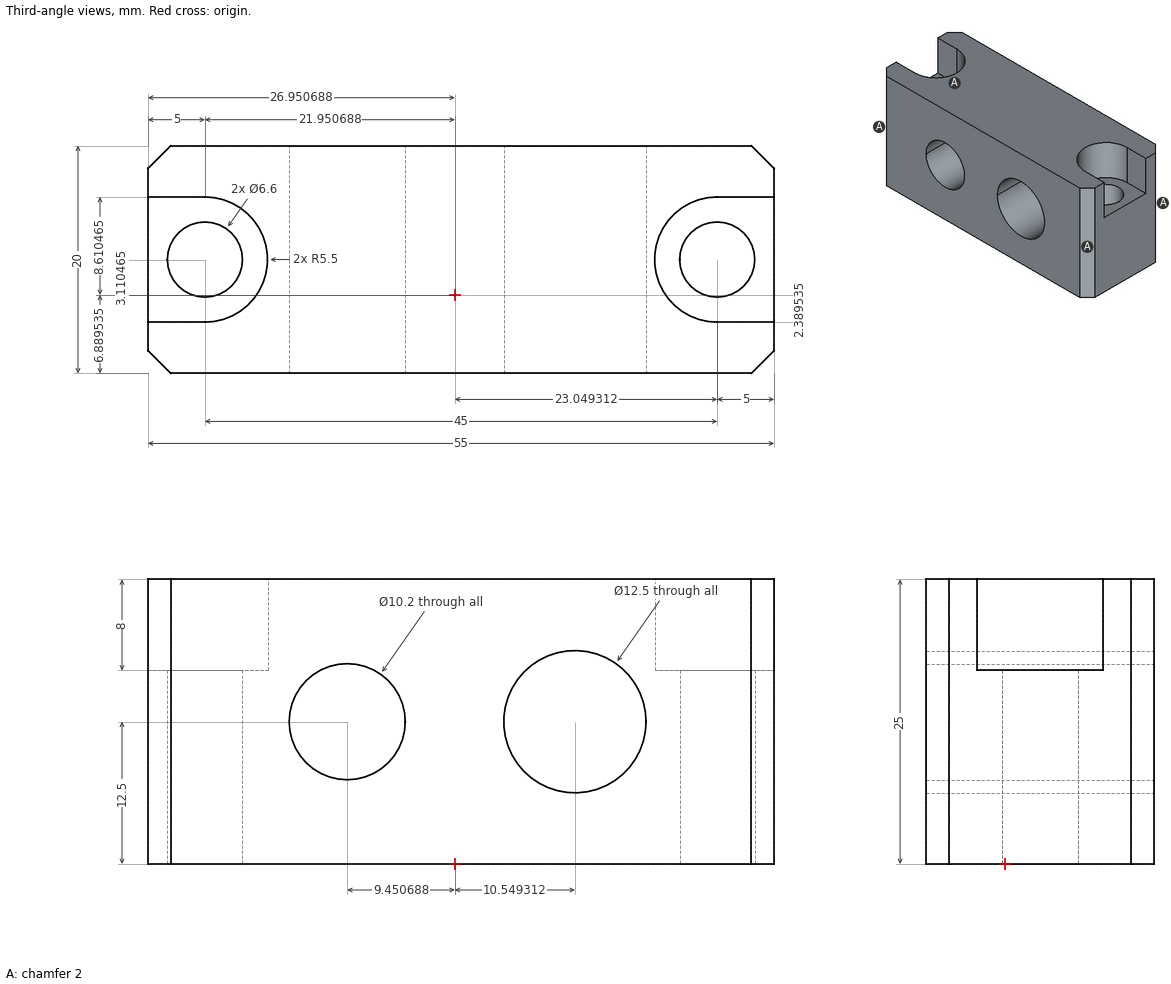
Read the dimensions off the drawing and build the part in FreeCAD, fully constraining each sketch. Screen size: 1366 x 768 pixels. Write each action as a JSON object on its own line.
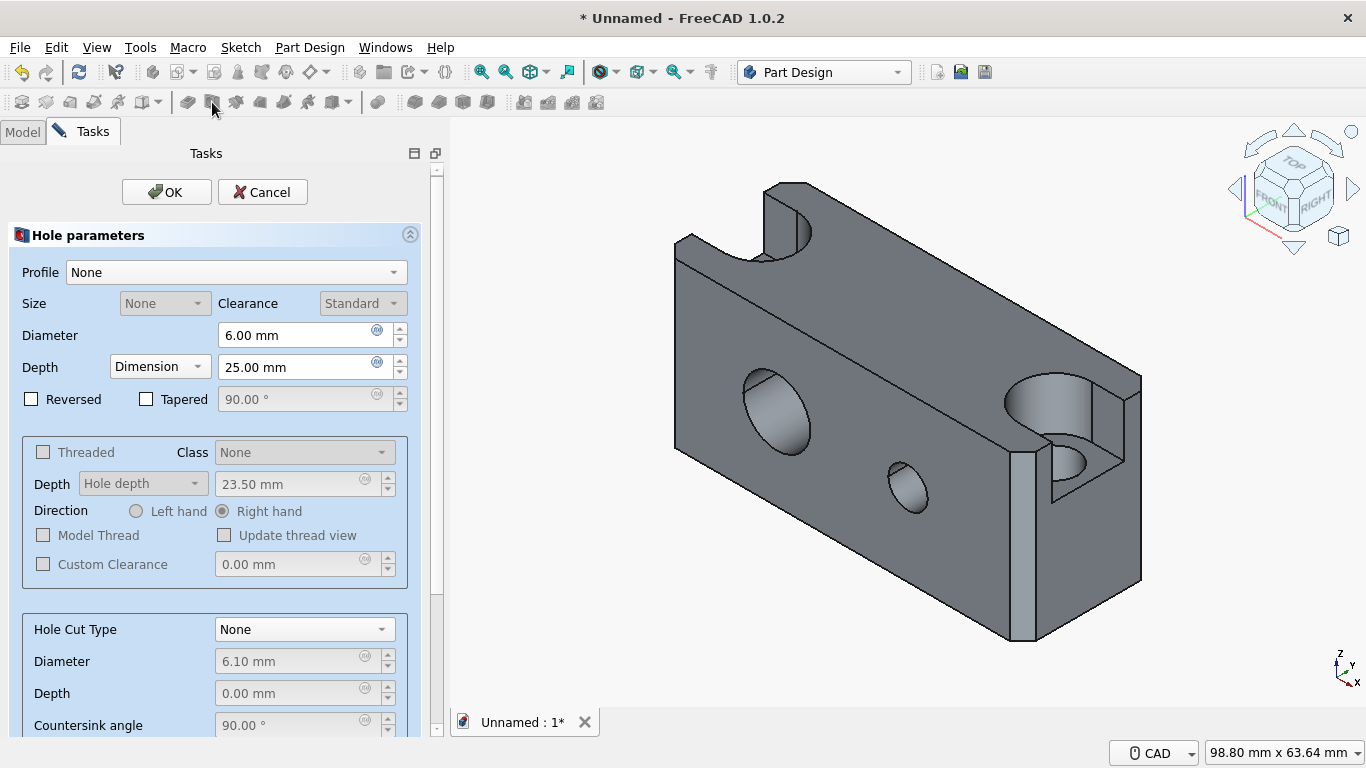
{"action": "triple_click", "coordinate": [305, 335]}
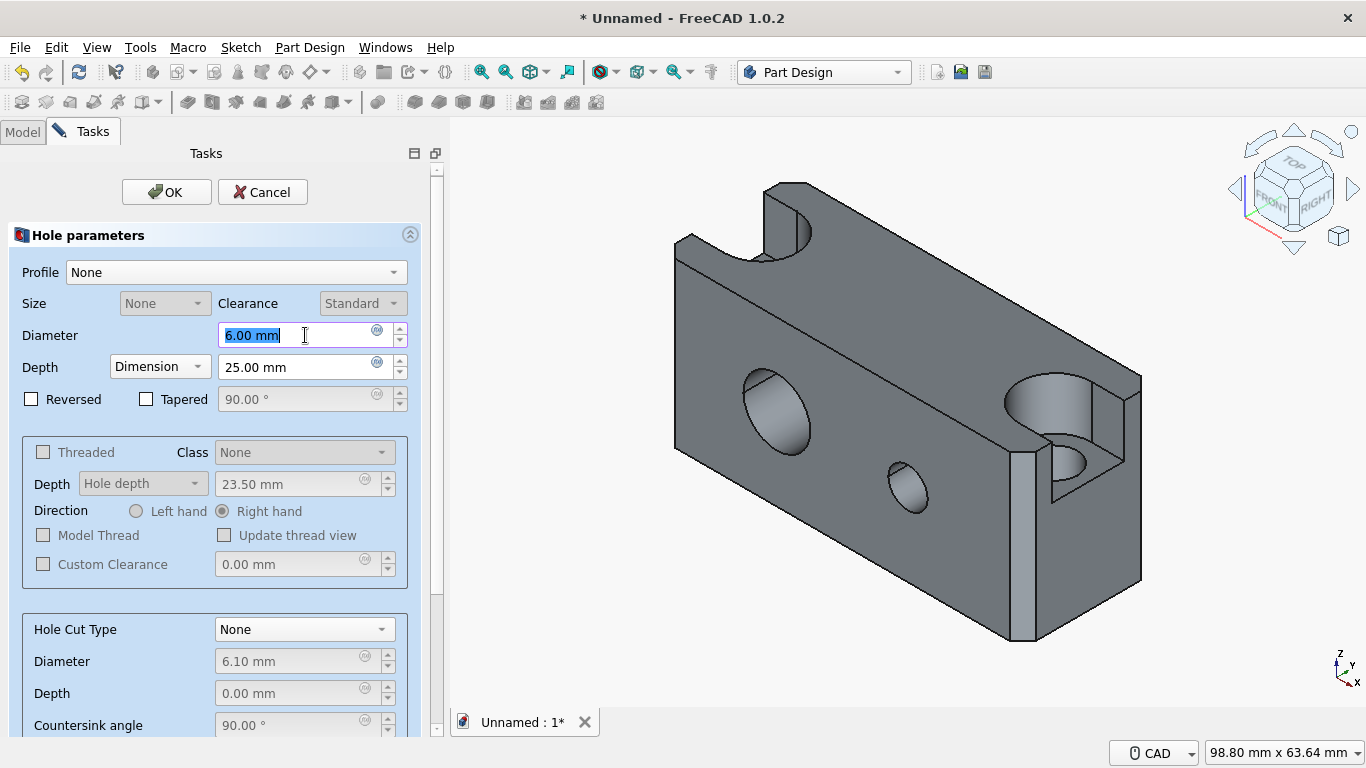
{"action": "type", "text": "12.5"}
{"action": "key", "text": "Tab"}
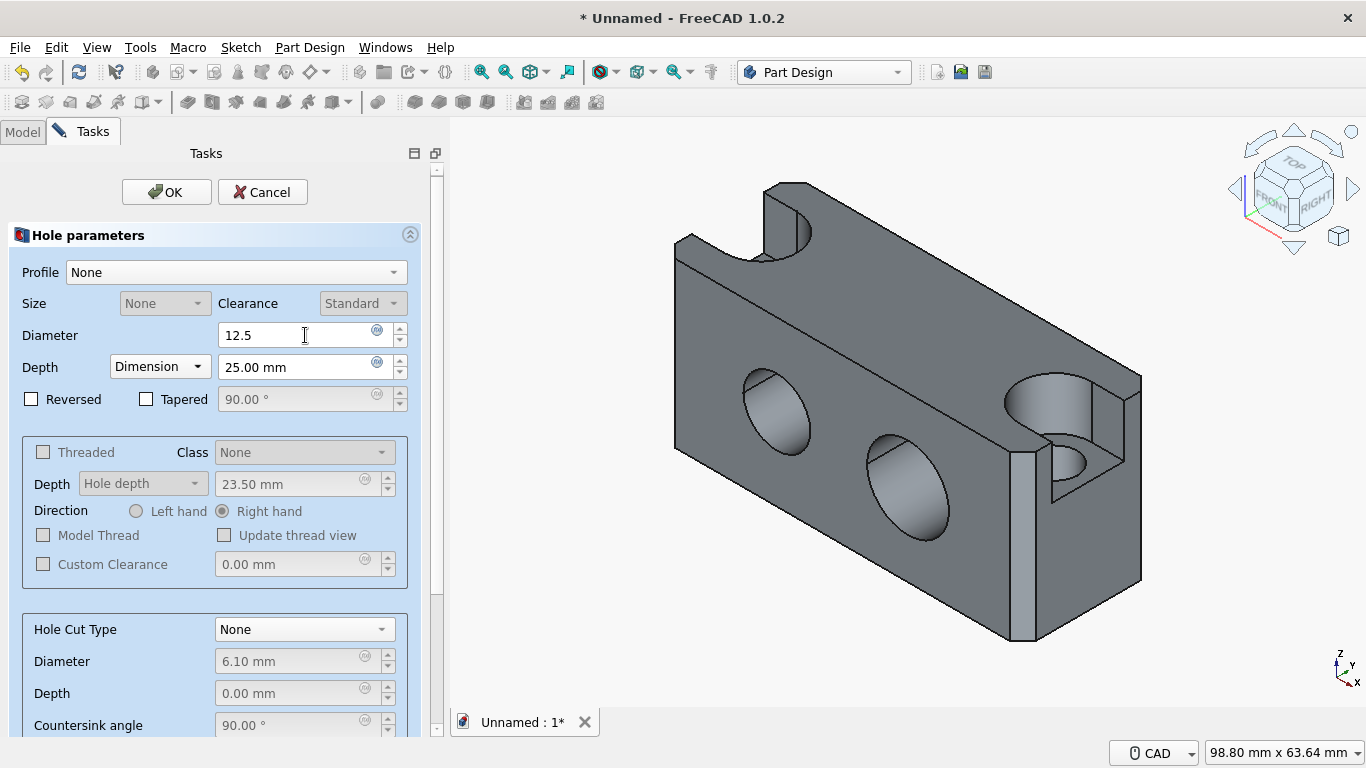
{"action": "left_click", "coordinate": [161, 366]}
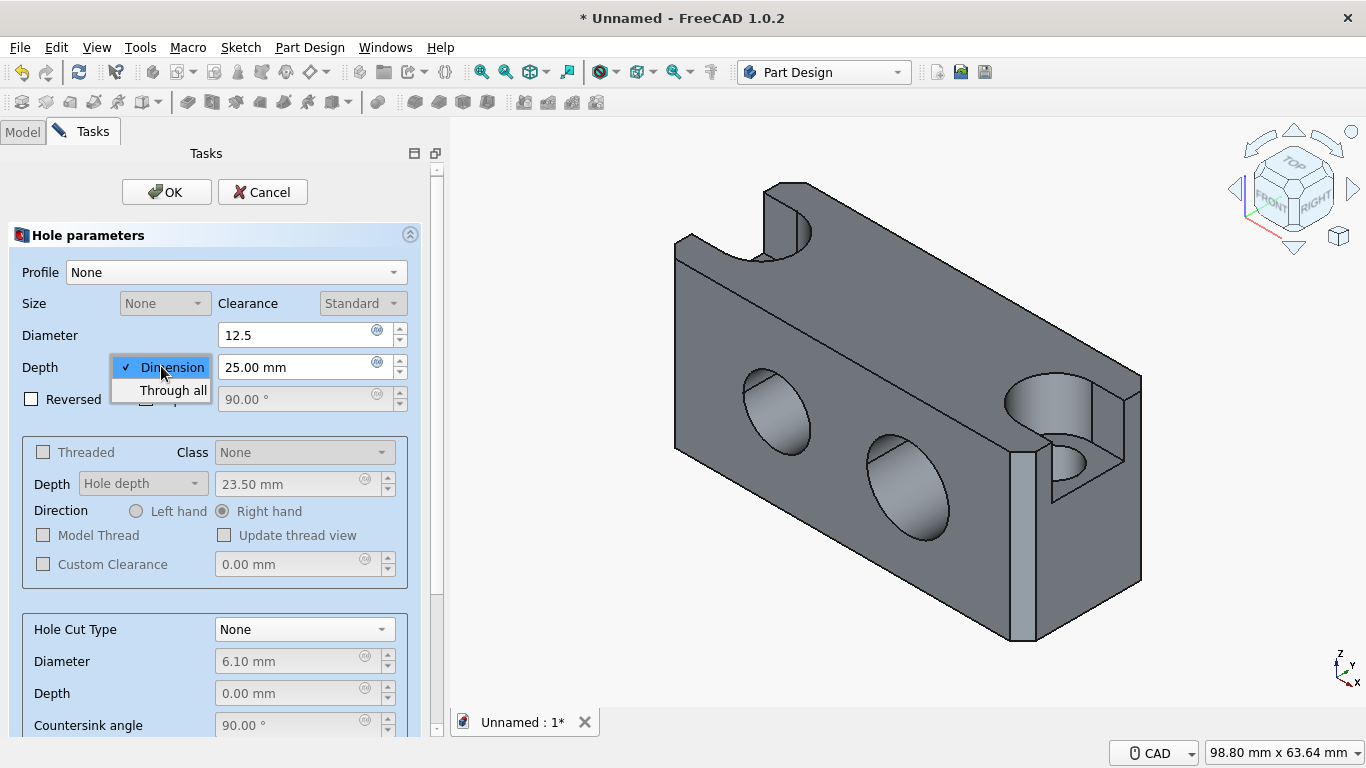
{"action": "left_click", "coordinate": [160, 390]}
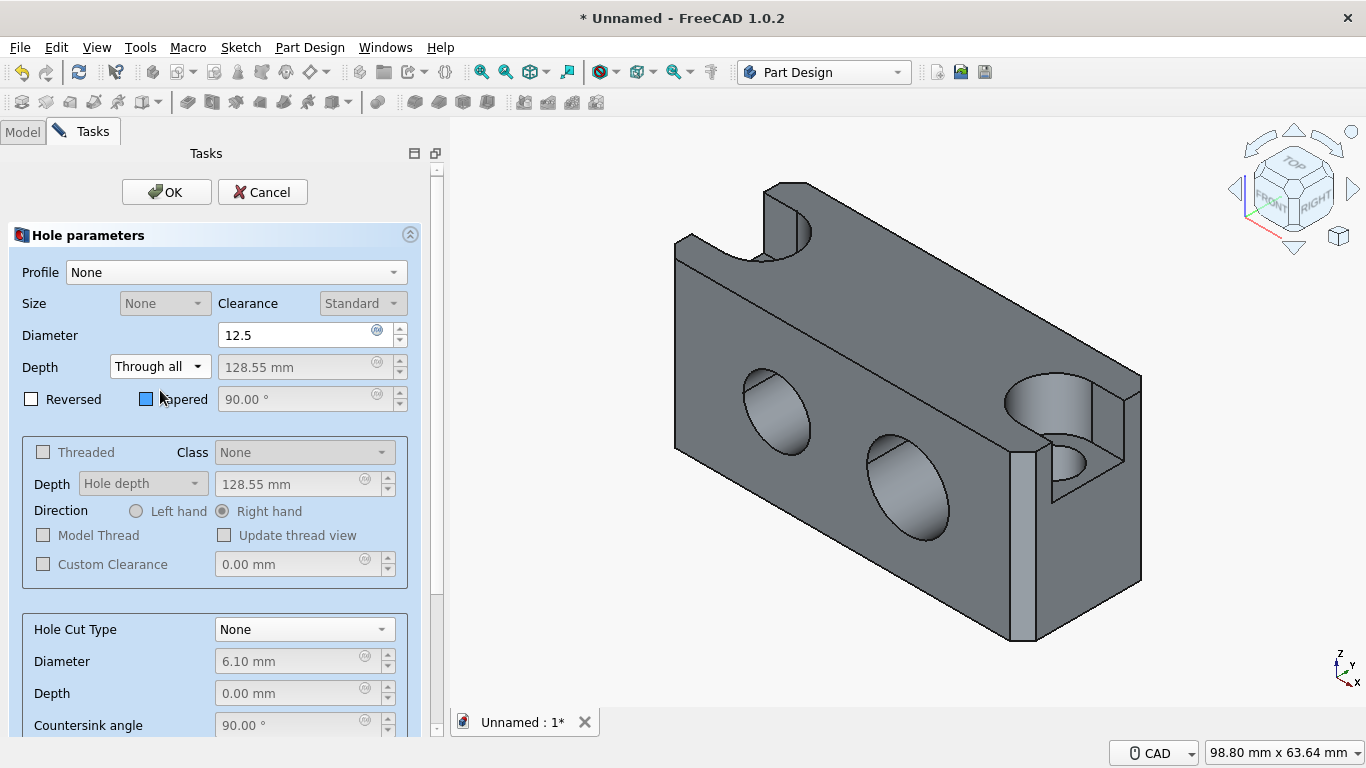
{"action": "left_click", "coordinate": [167, 192]}